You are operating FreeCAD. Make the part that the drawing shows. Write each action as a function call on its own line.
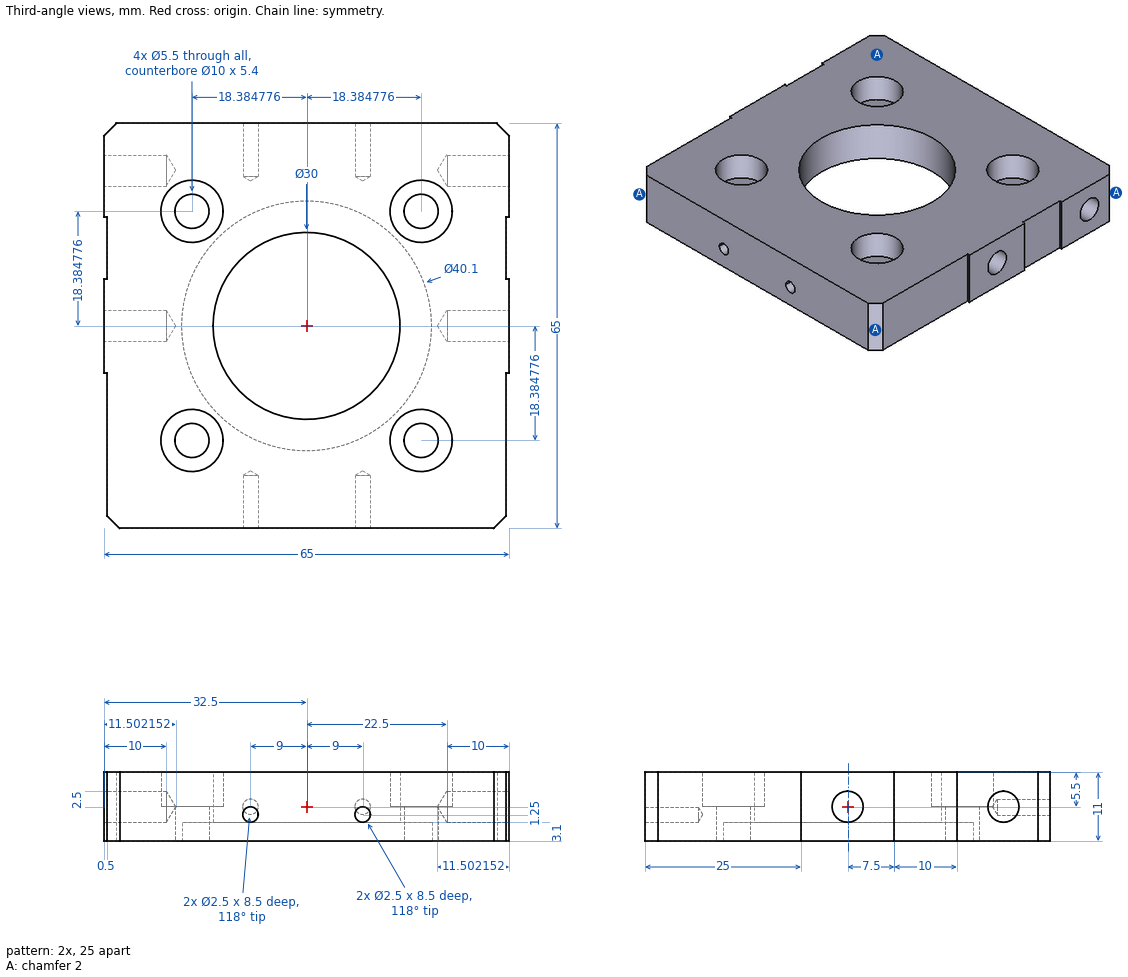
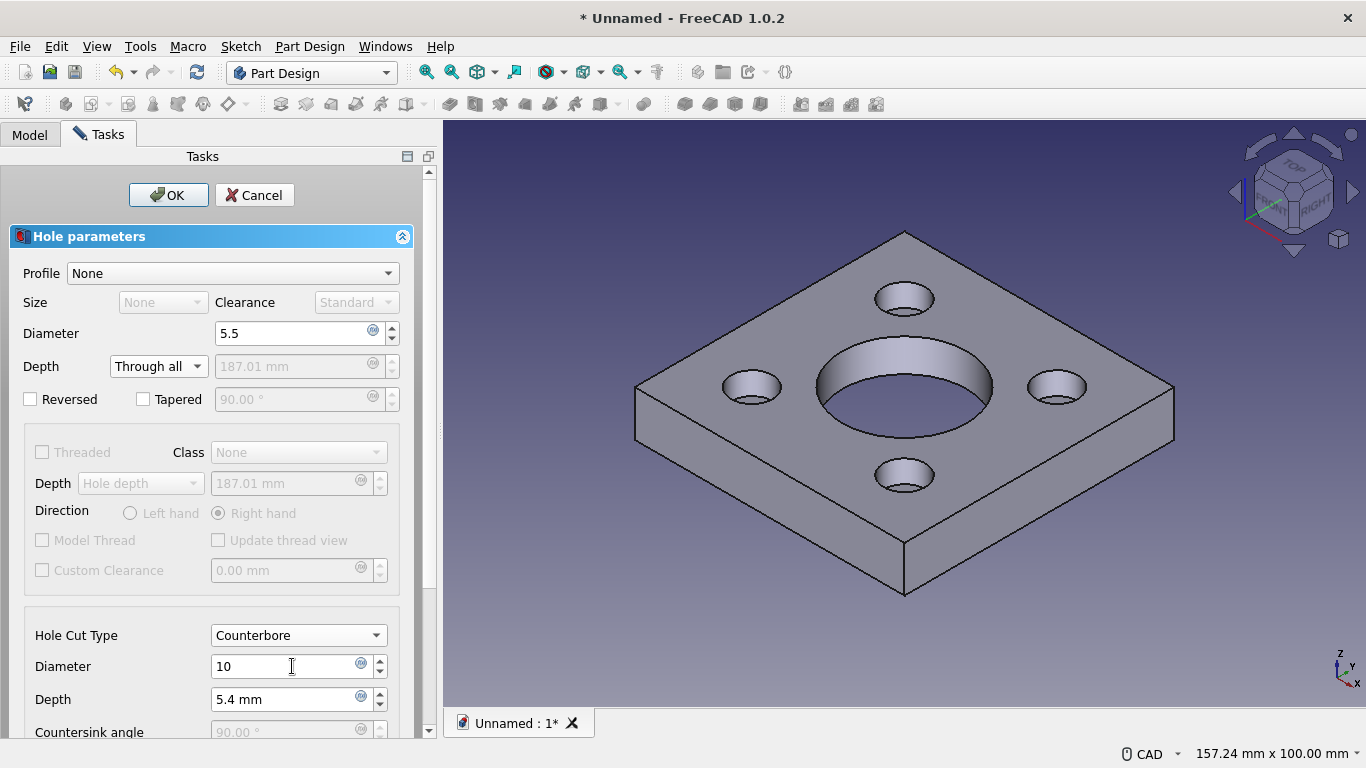
click(169, 195)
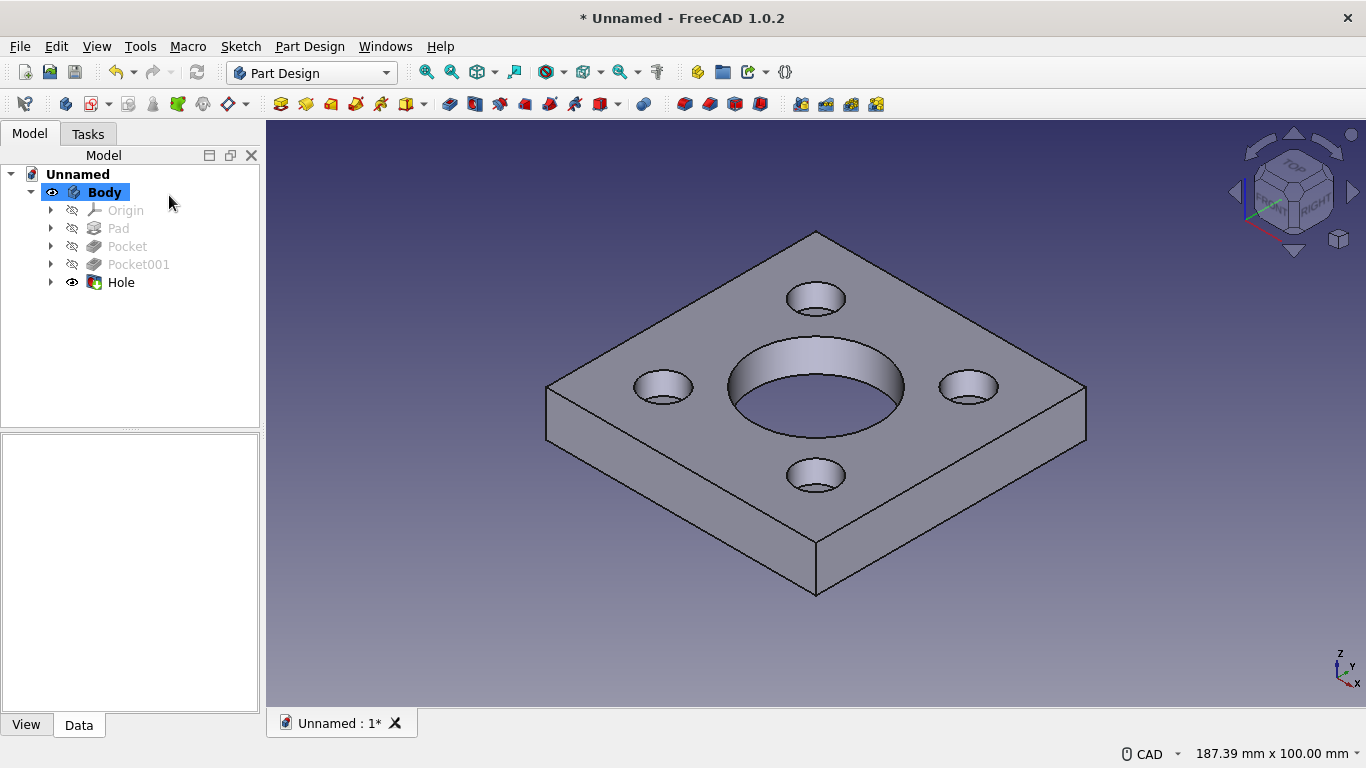
click(90, 104)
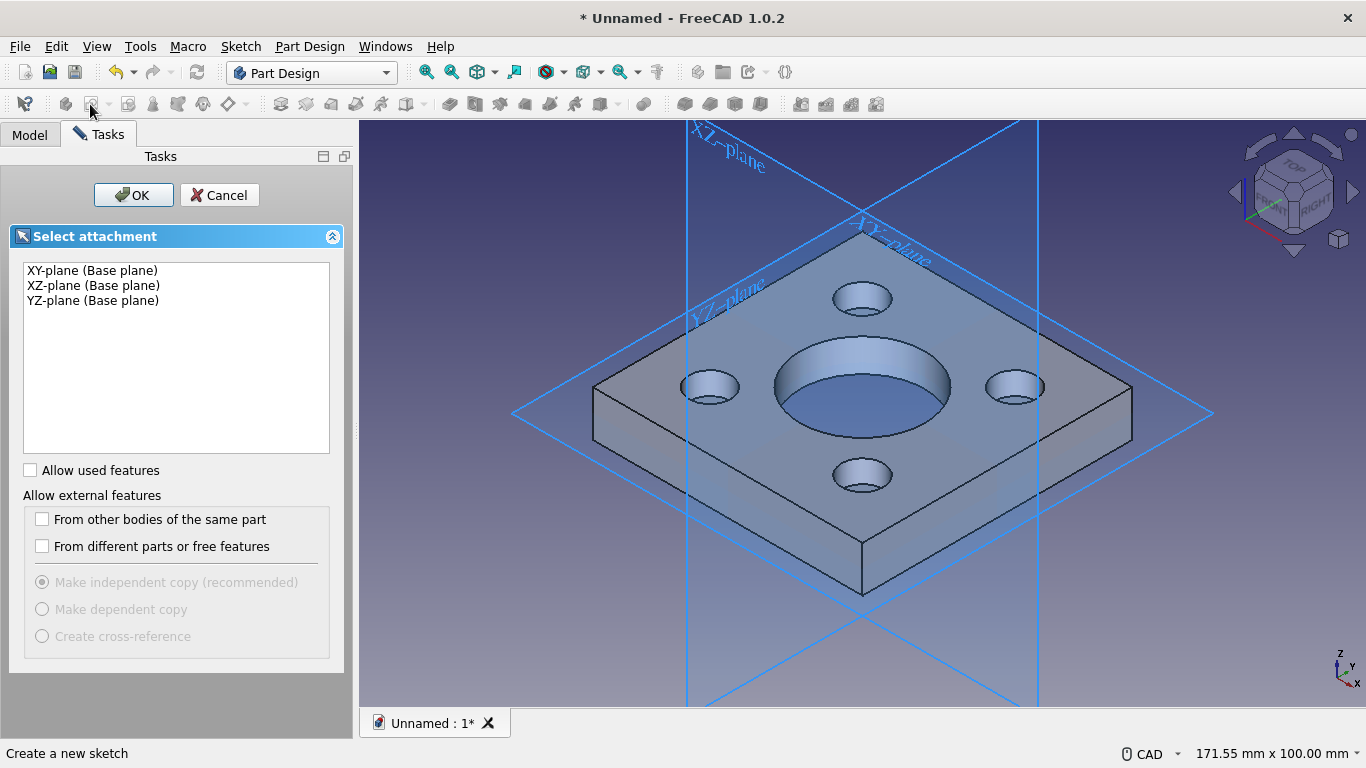
click(84, 286)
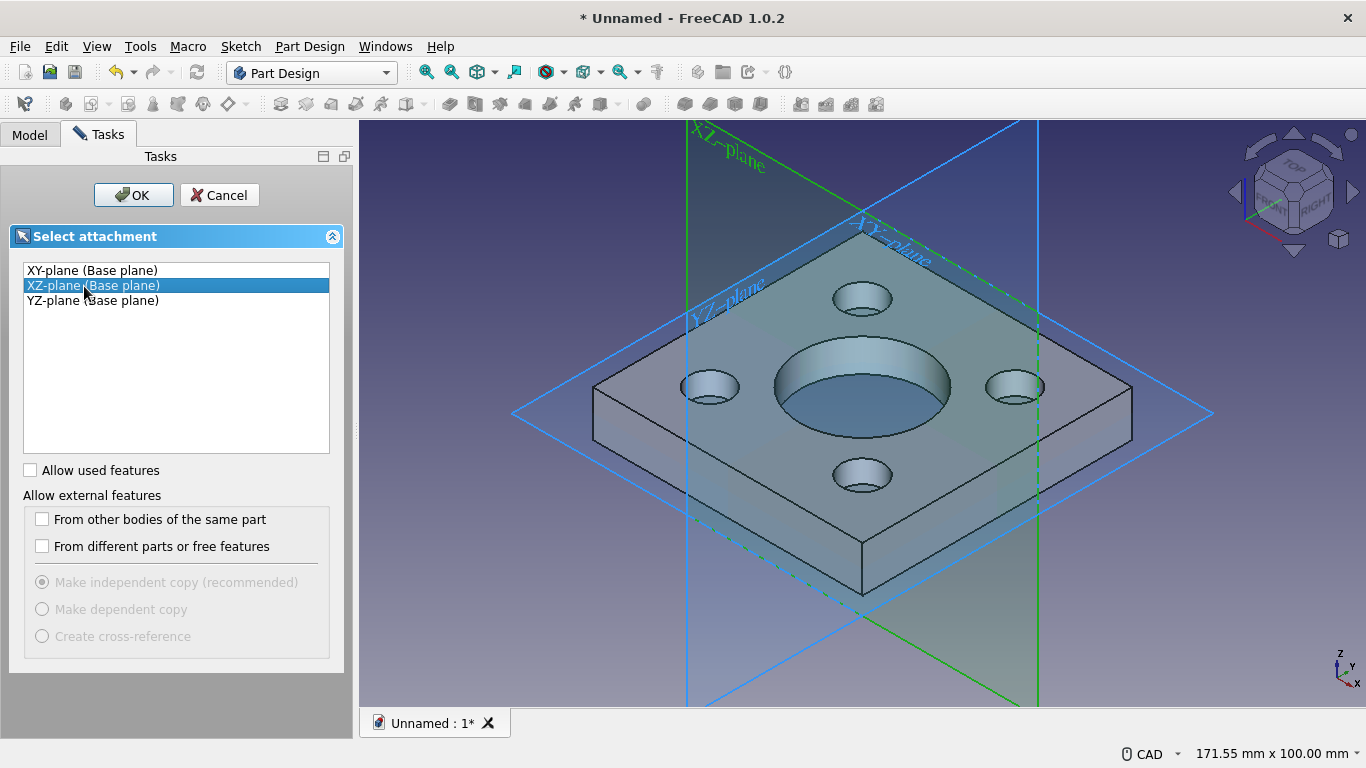
click(134, 195)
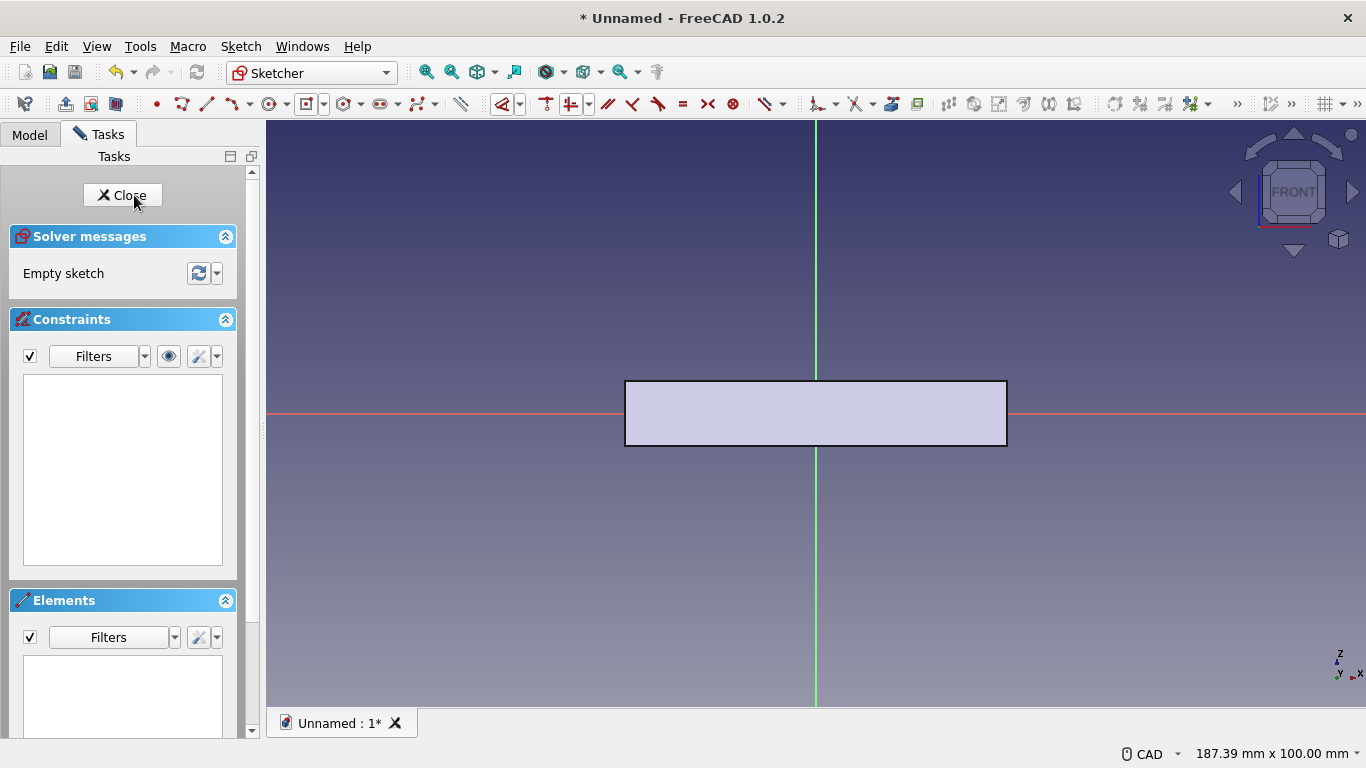
click(116, 104)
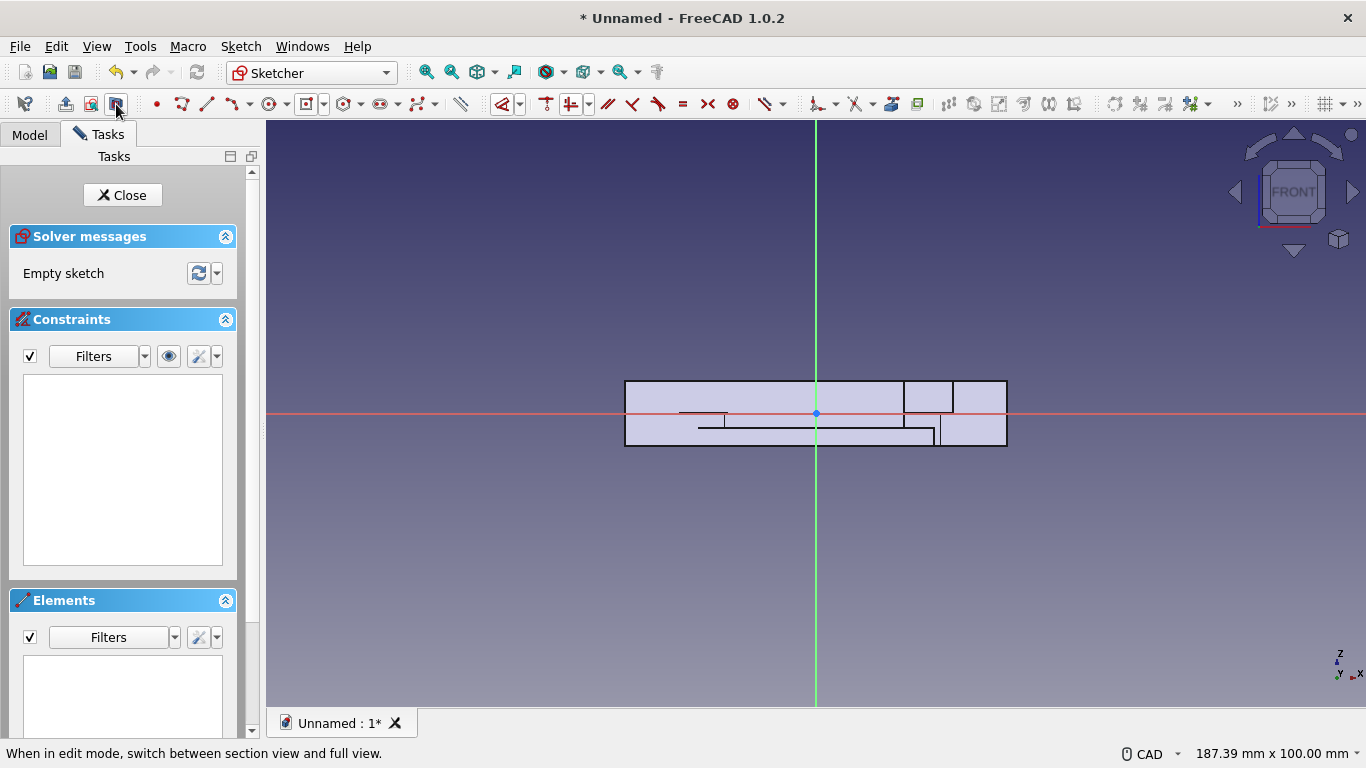
scroll(648, 405, up, 11)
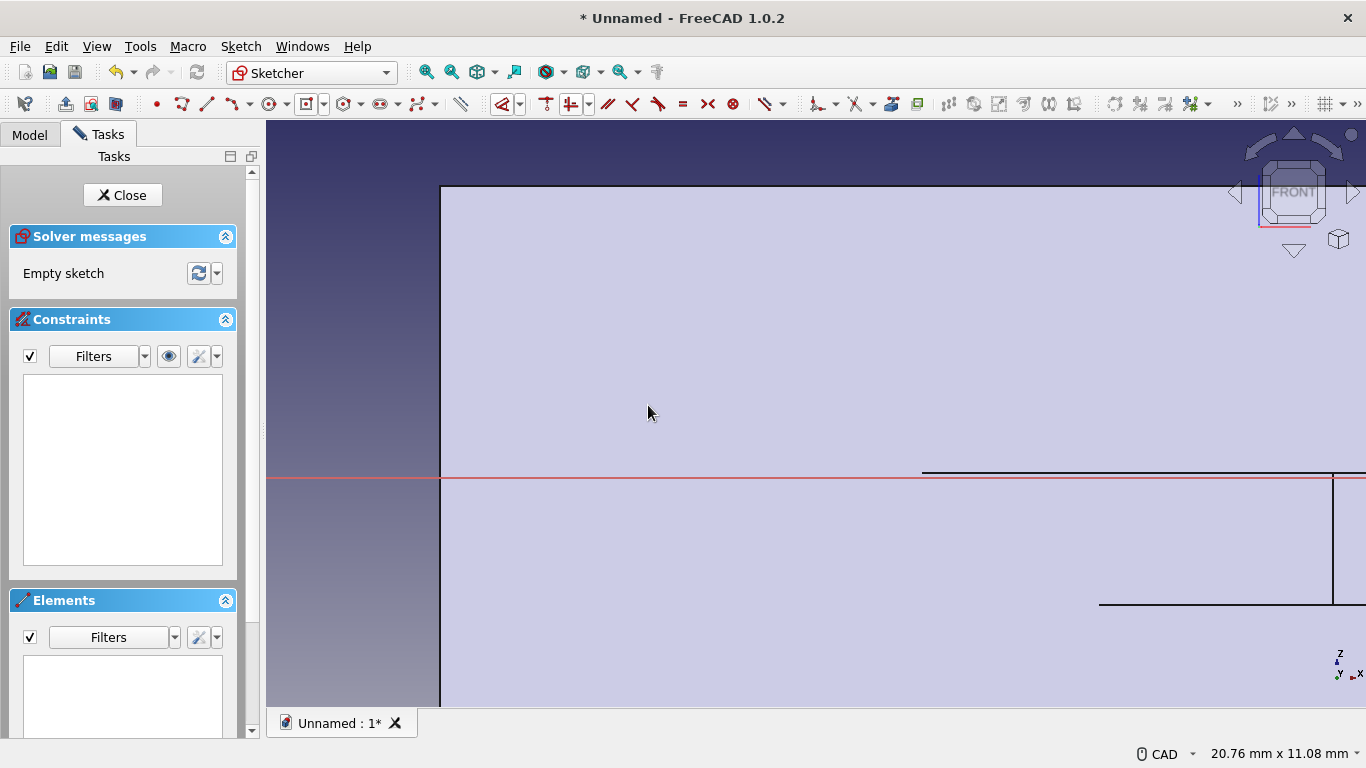
click(182, 104)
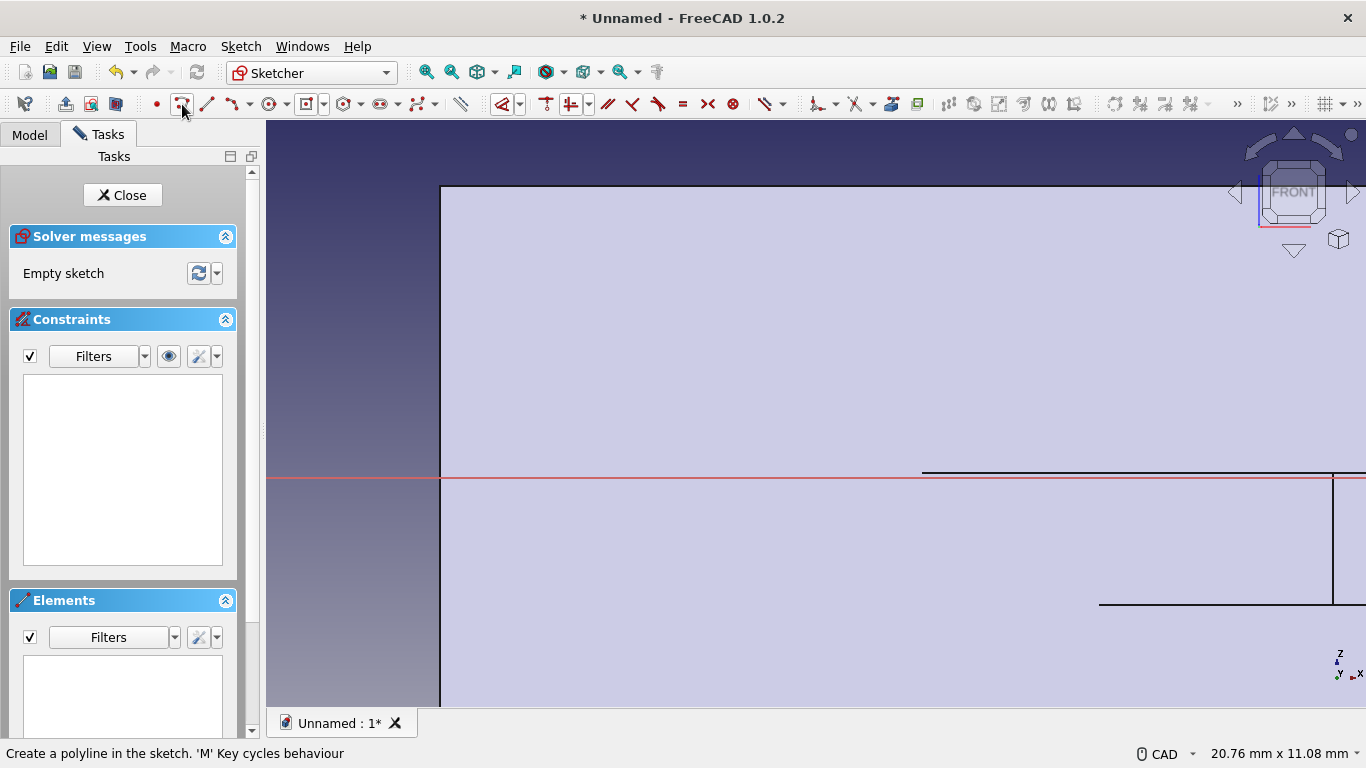
click(1049, 478)
click(440, 469)
click(440, 345)
click(969, 345)
click(1049, 478)
key(Escape)
key(Escape)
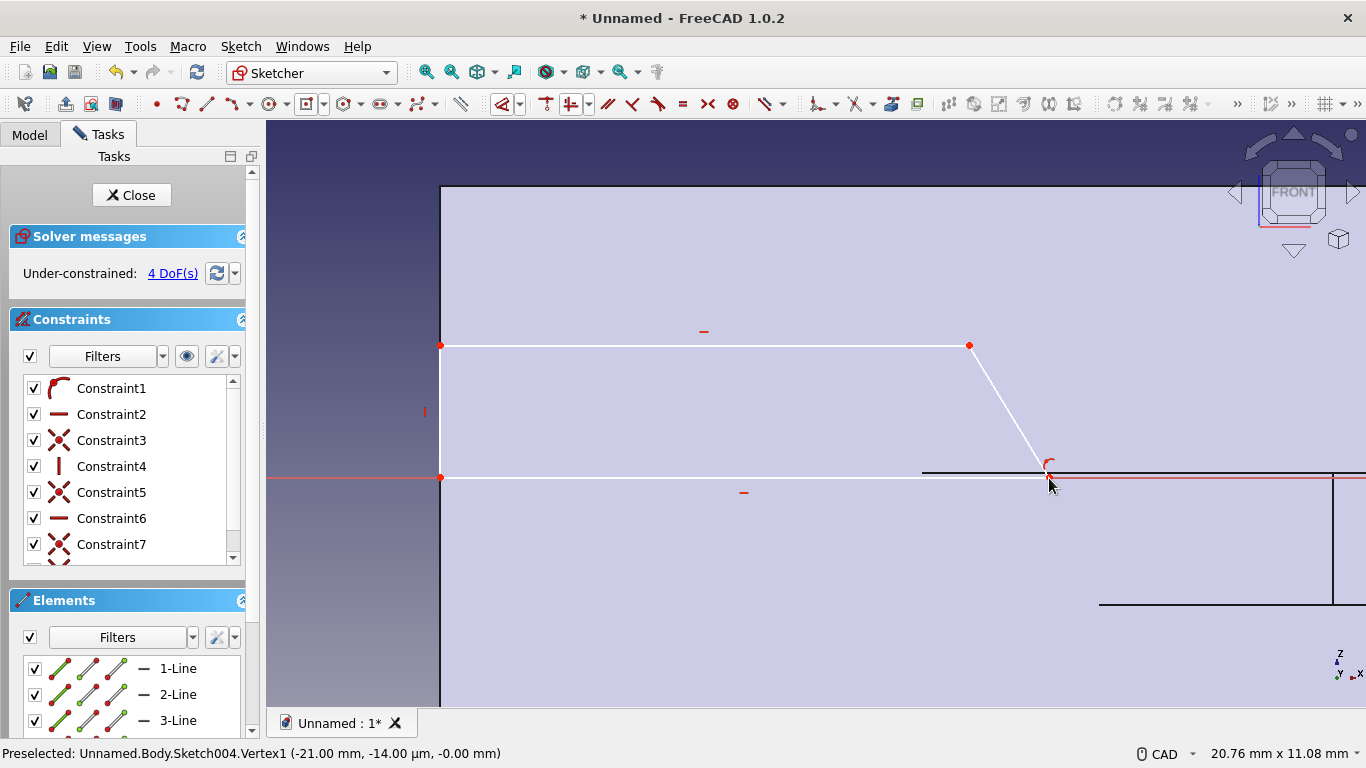
click(599, 346)